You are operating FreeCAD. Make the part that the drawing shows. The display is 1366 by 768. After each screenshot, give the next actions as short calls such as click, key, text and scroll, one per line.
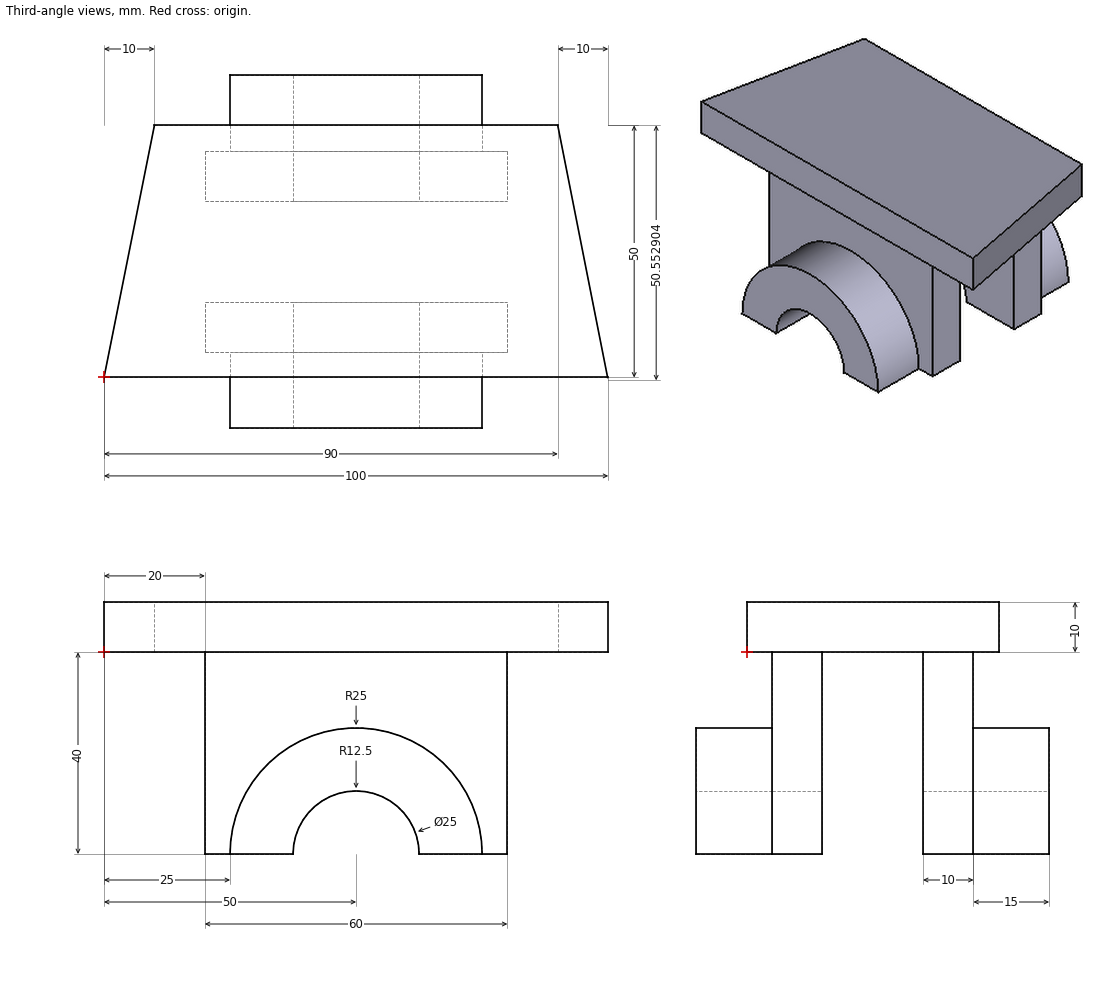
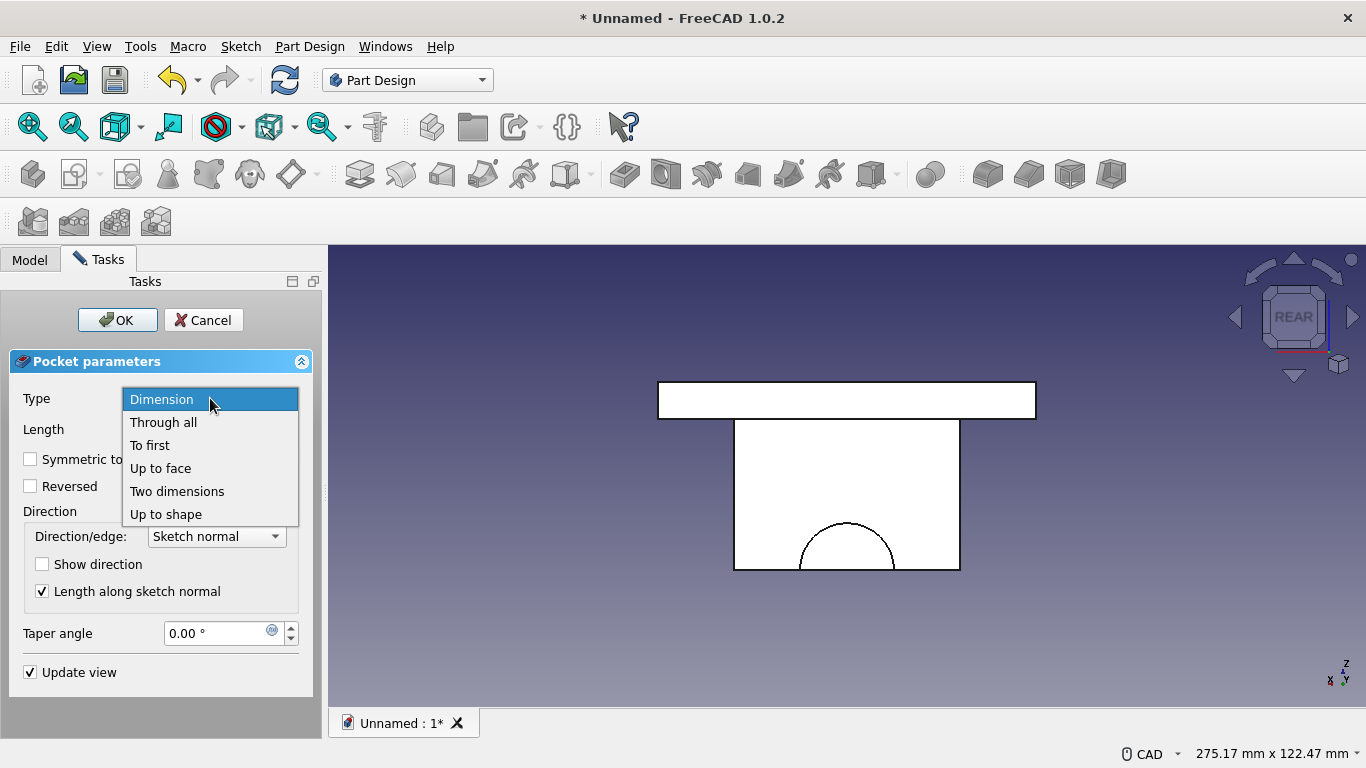
click(208, 422)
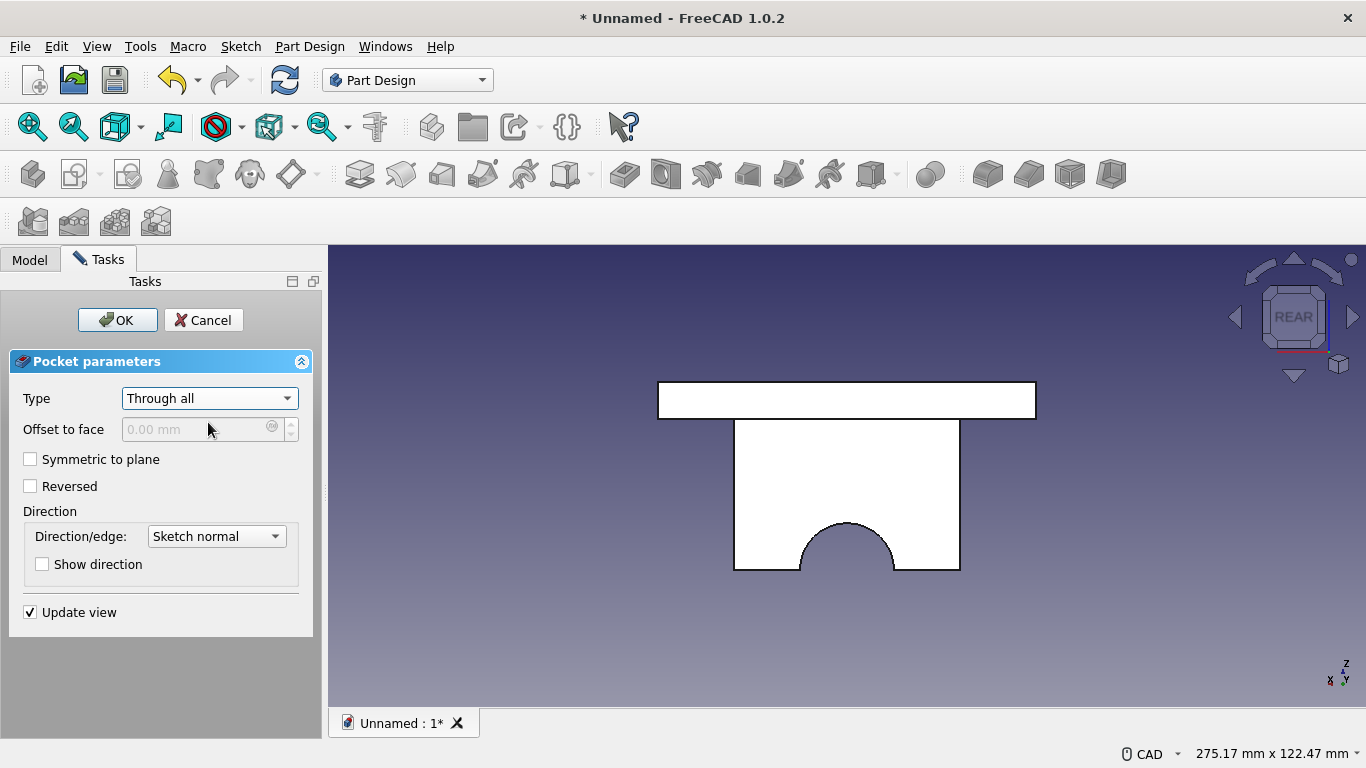
click(118, 320)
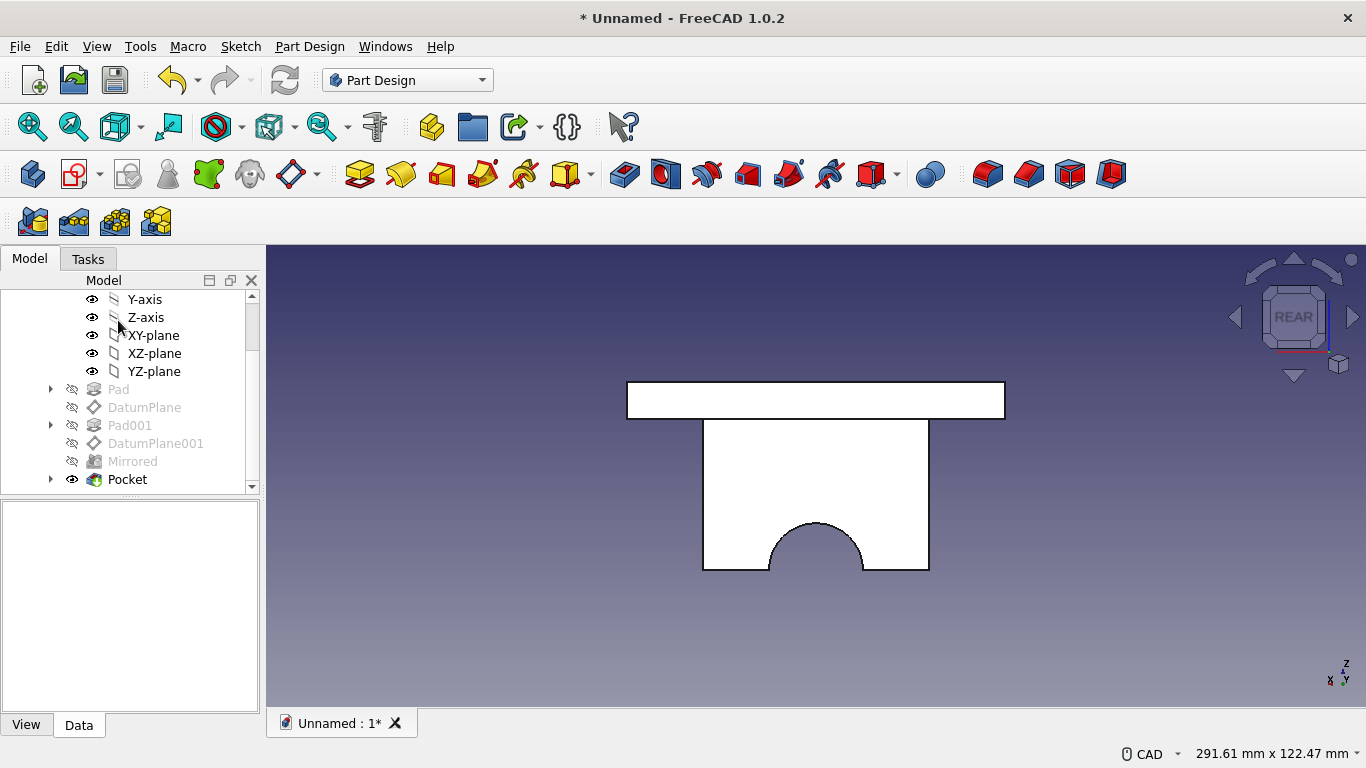
key(v)
key(f)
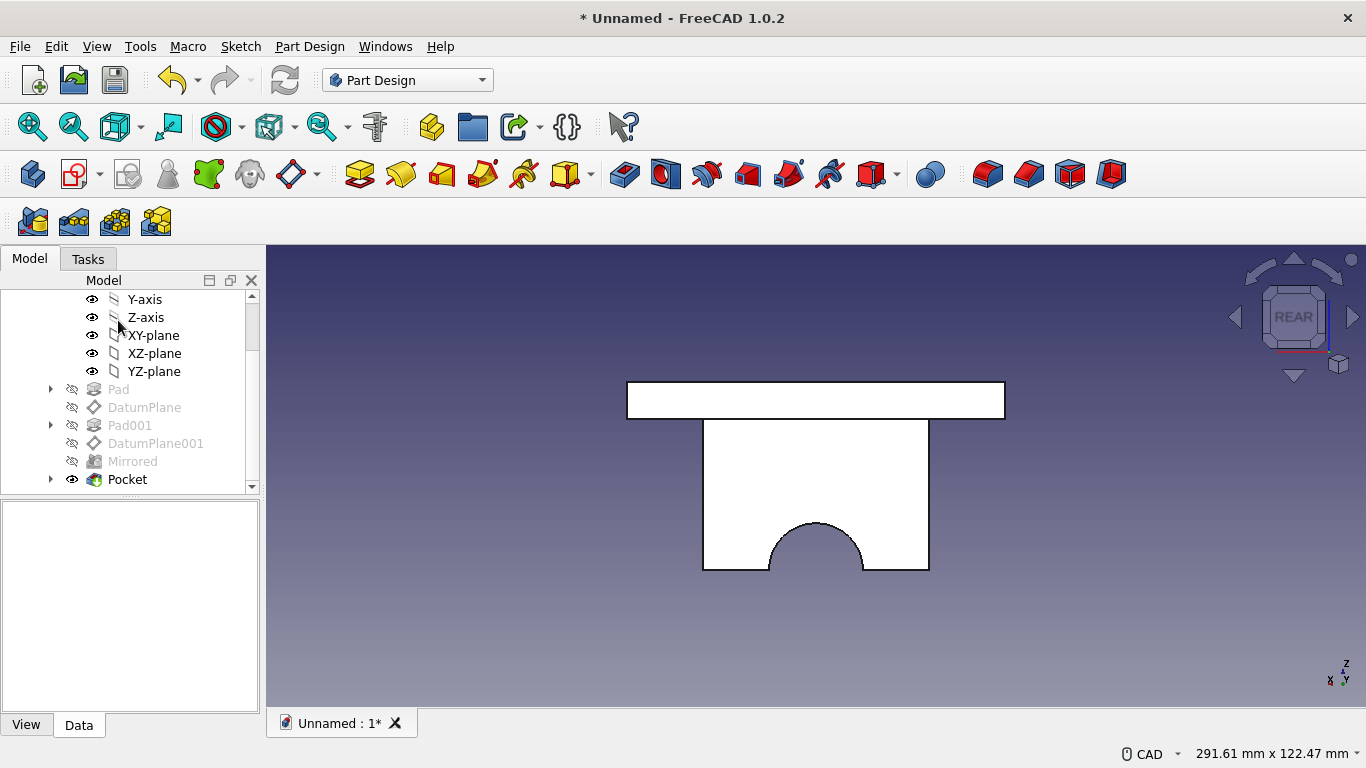
scroll(161, 385, down, 3)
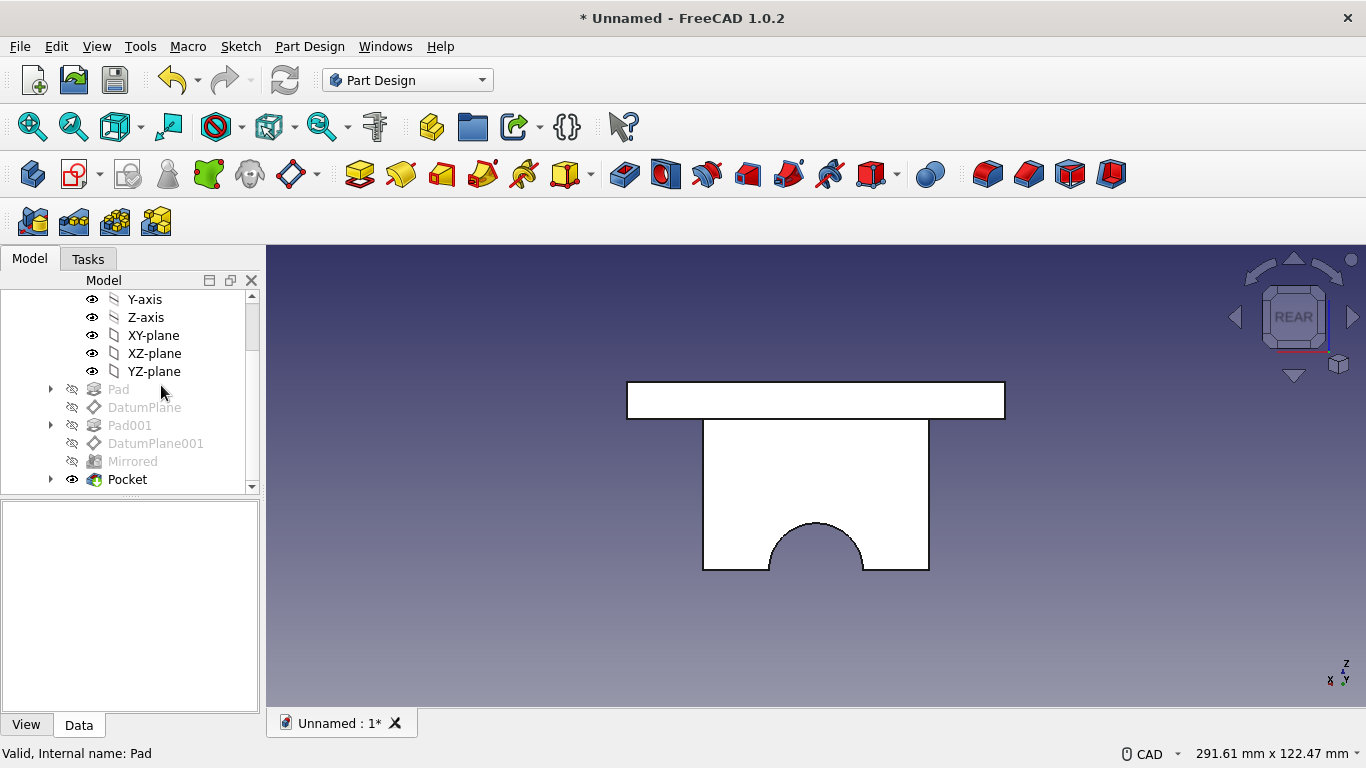
scroll(161, 385, up, 15)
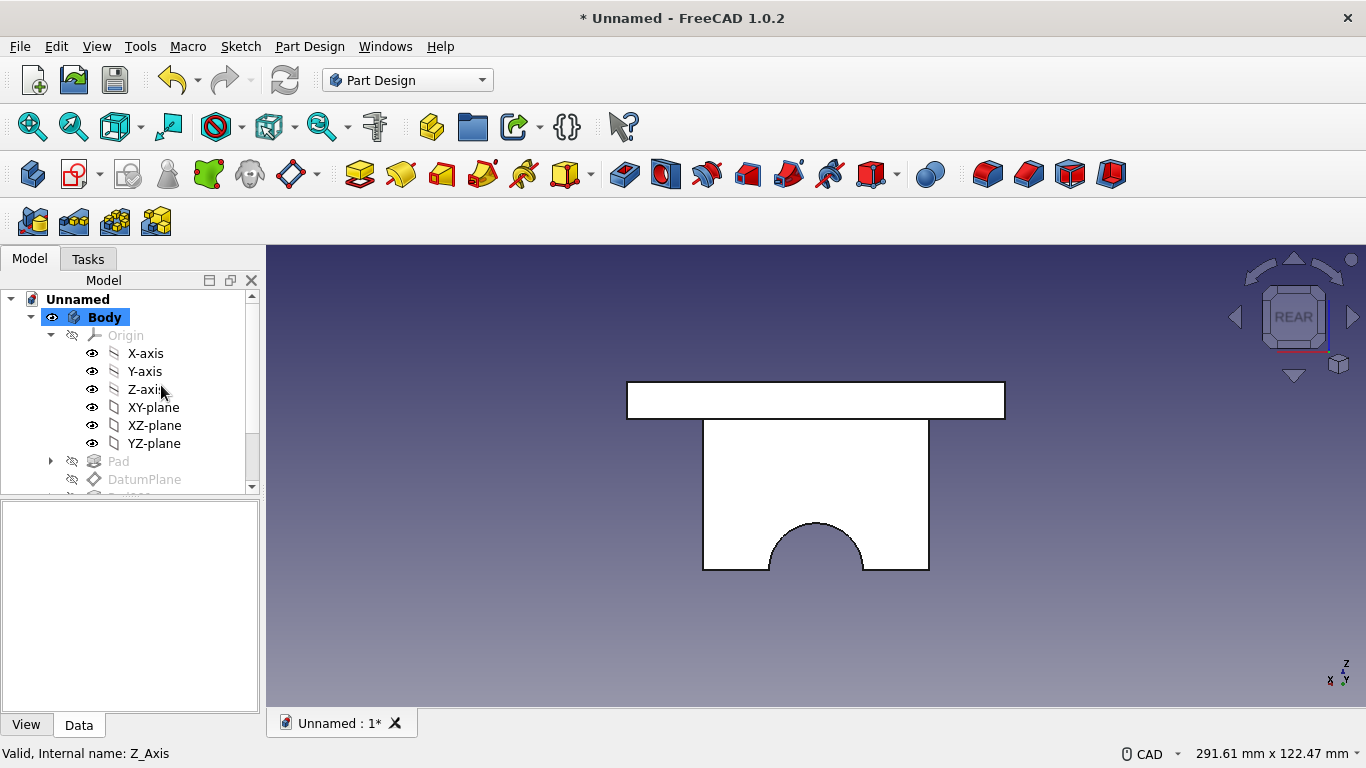
click(137, 425)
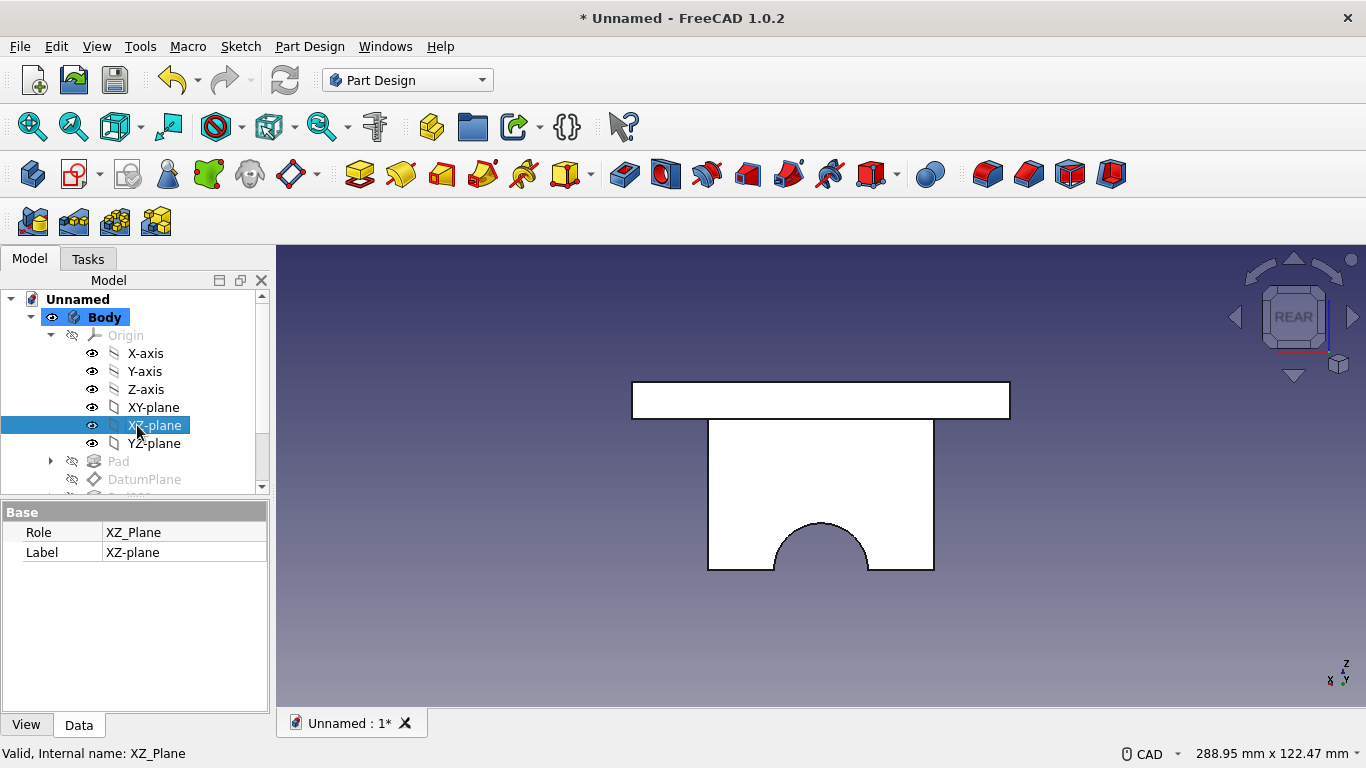
click(290, 174)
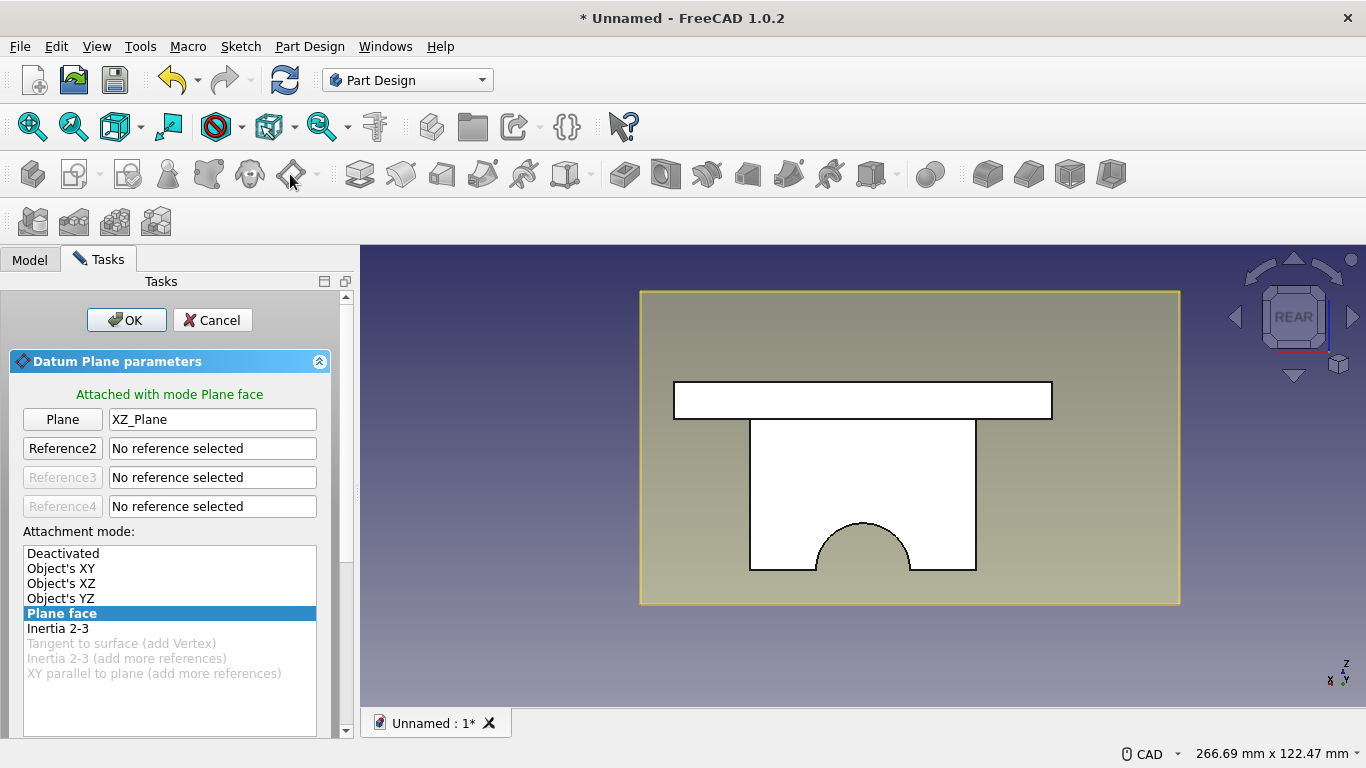
scroll(346, 514, down, 4)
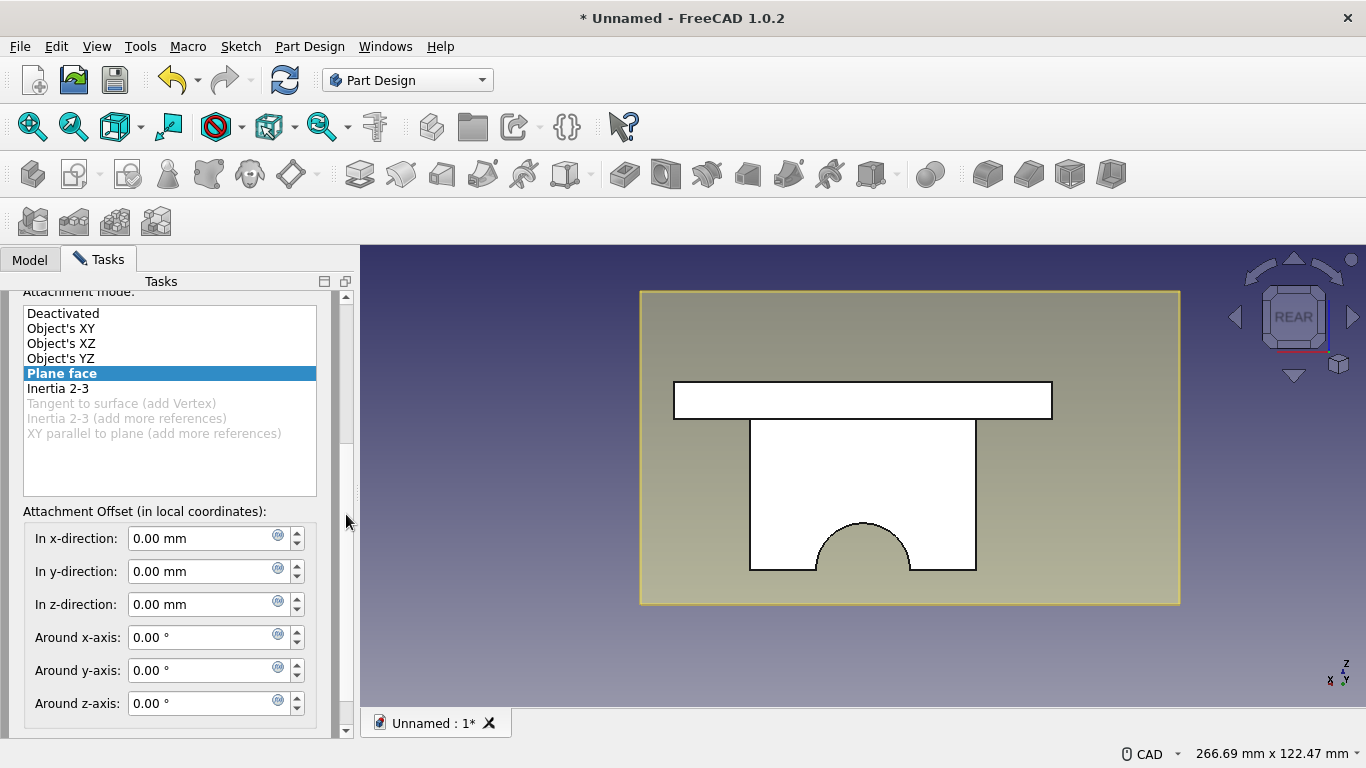
triple_click(210, 604)